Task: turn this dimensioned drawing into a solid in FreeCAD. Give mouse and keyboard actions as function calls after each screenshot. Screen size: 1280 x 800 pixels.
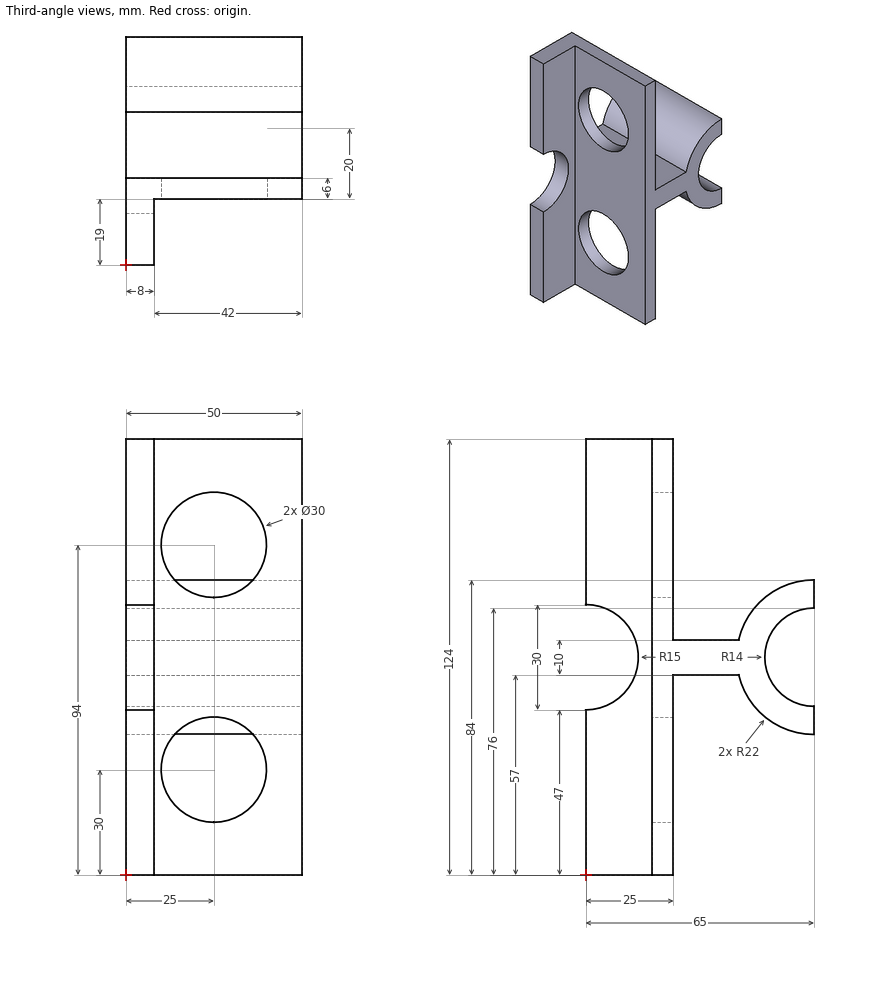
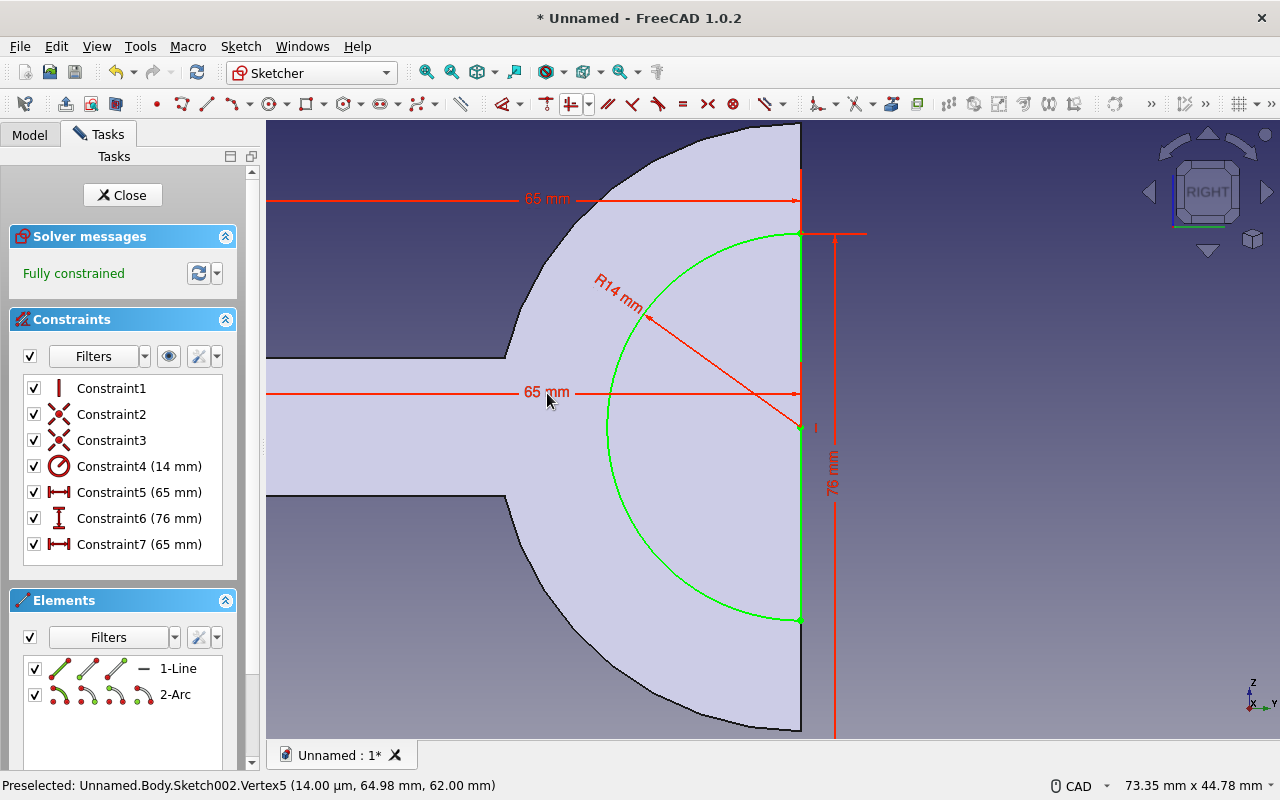
click(123, 195)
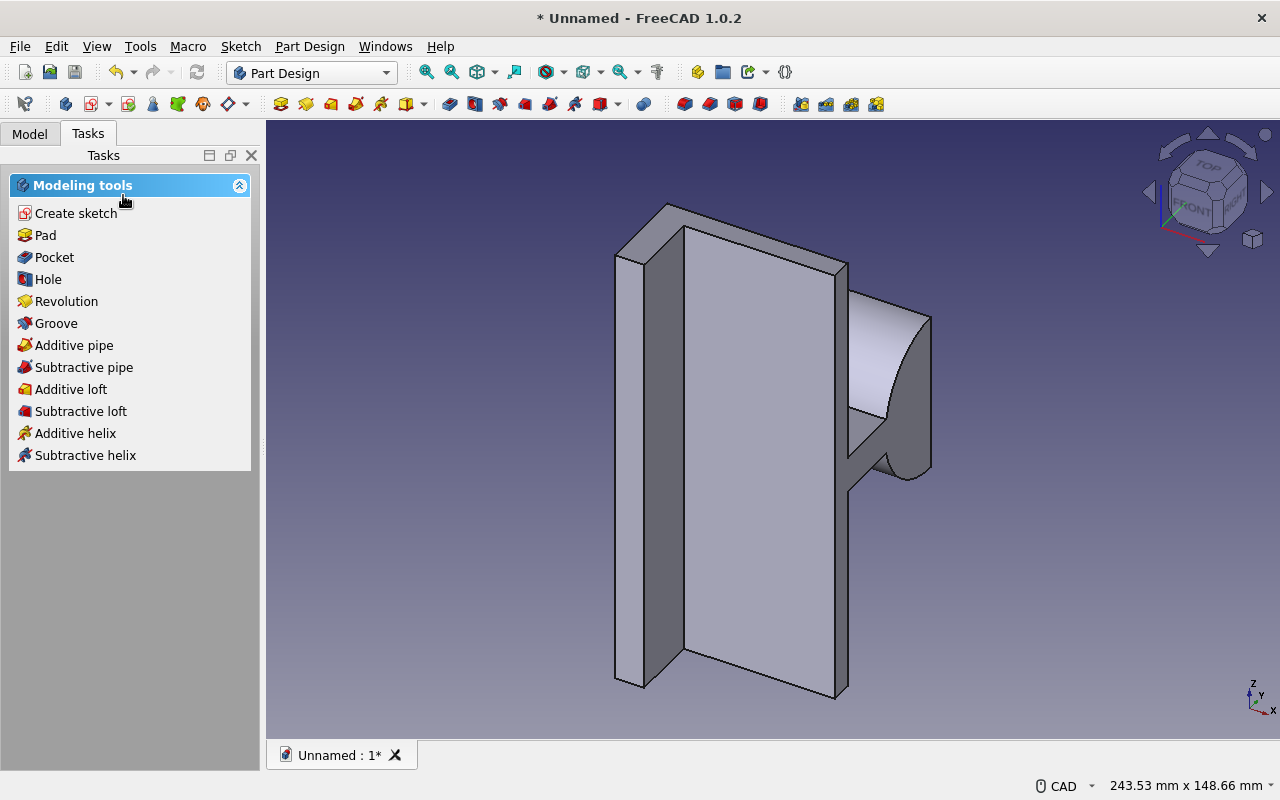
click(450, 104)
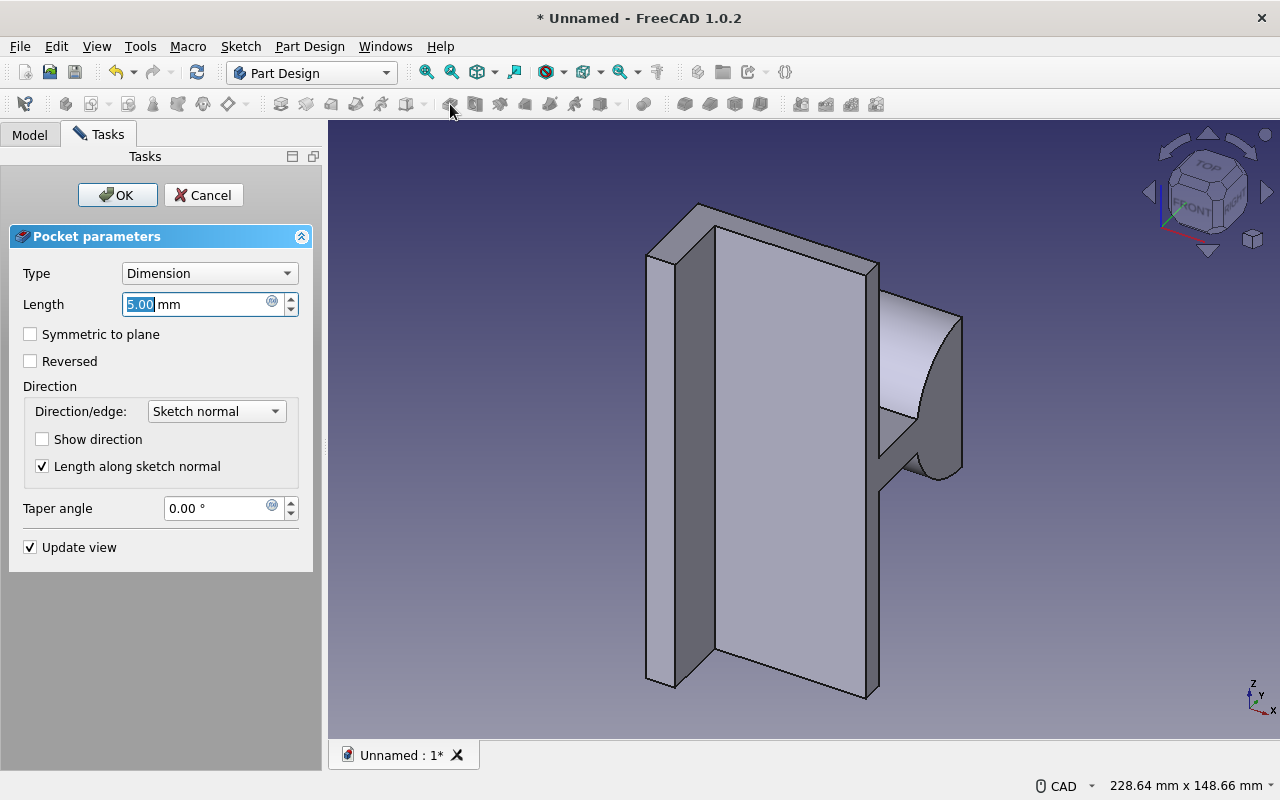
text(50)
key(Tab)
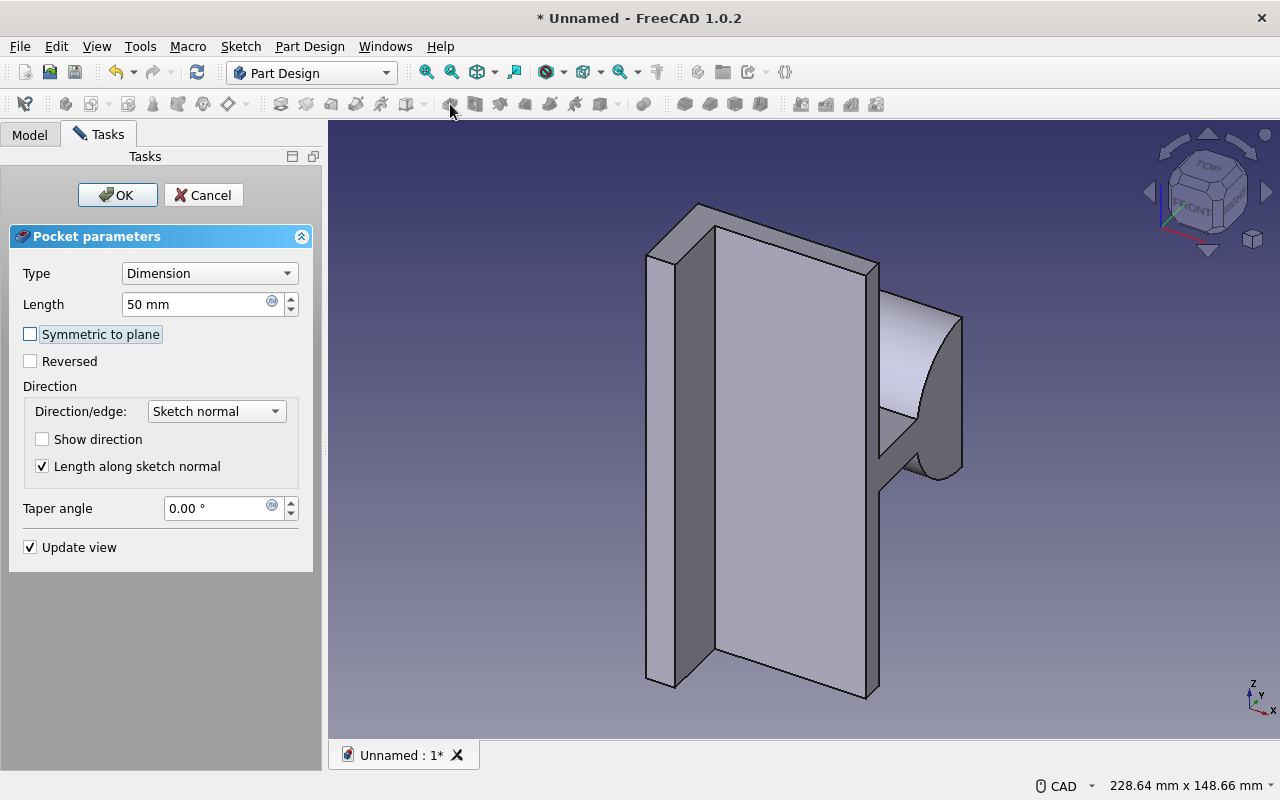
click(31, 361)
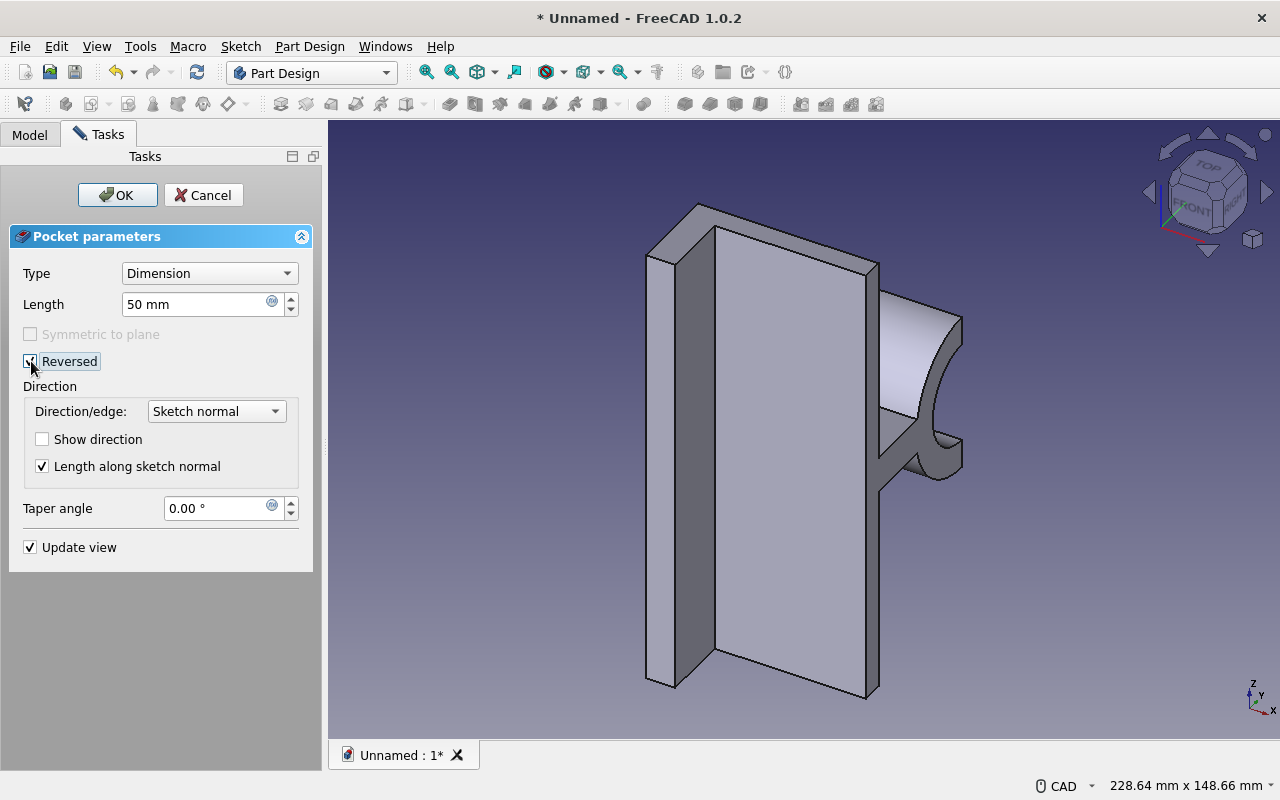
click(118, 195)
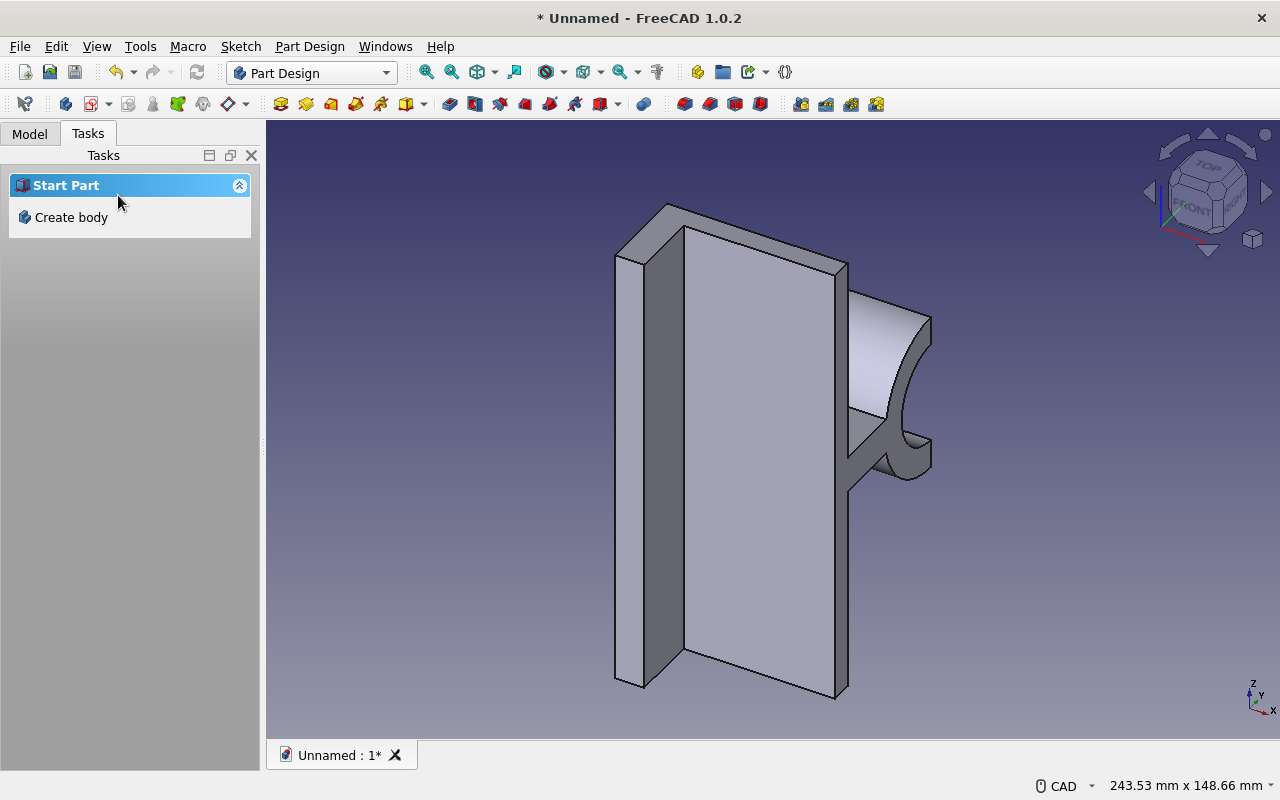
click(90, 104)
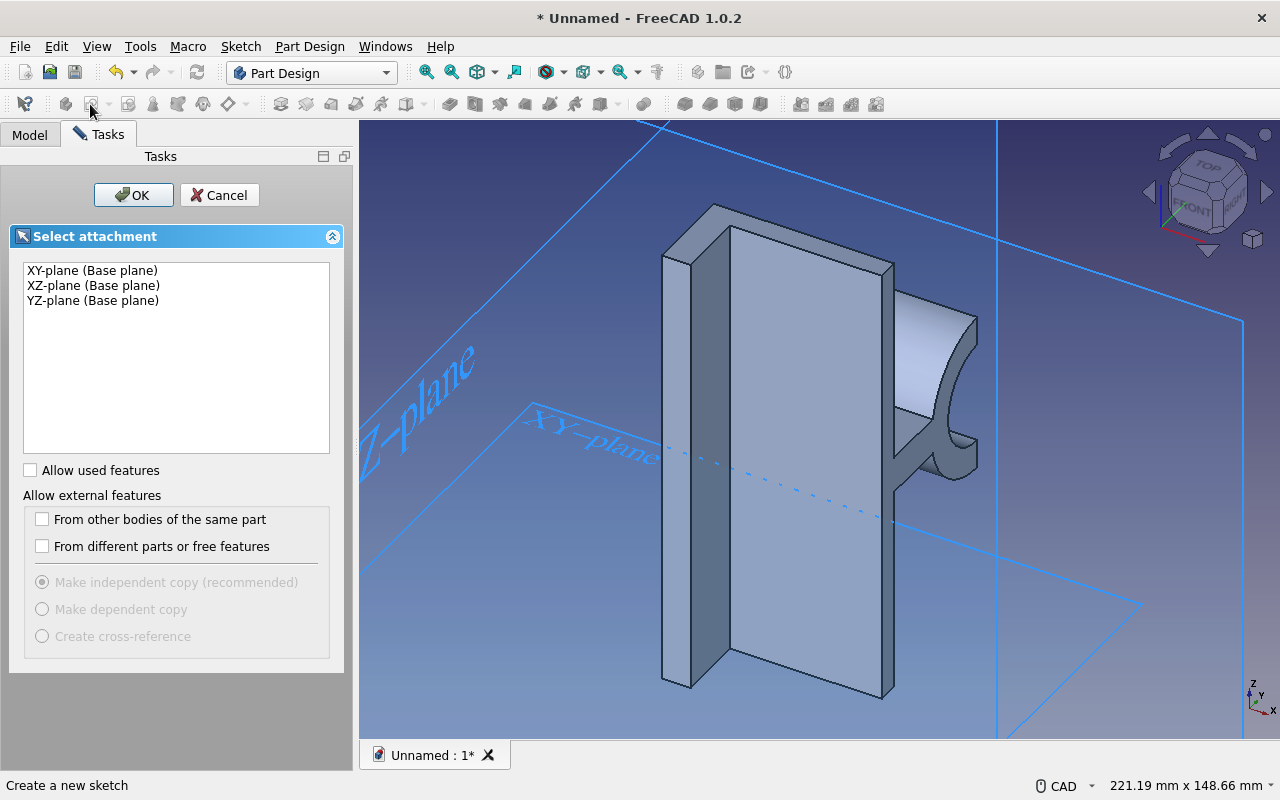
click(84, 300)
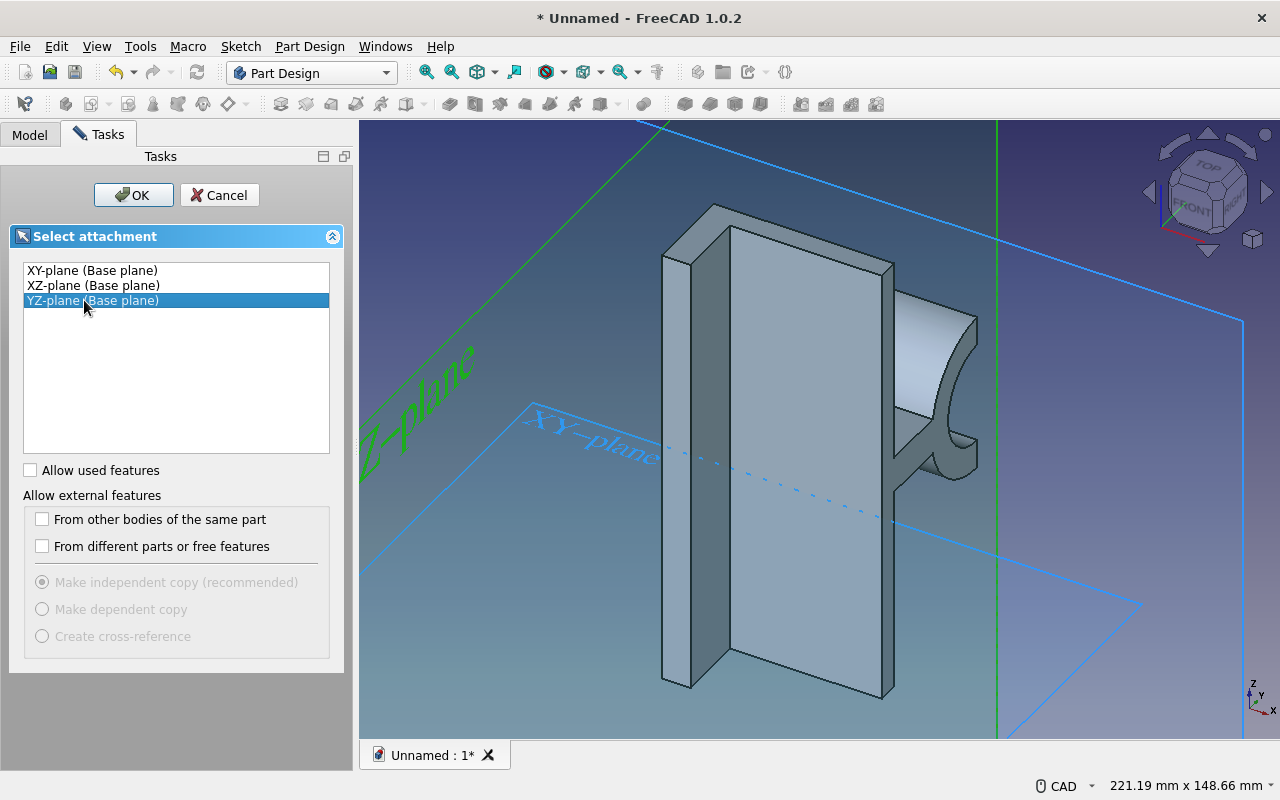
click(134, 195)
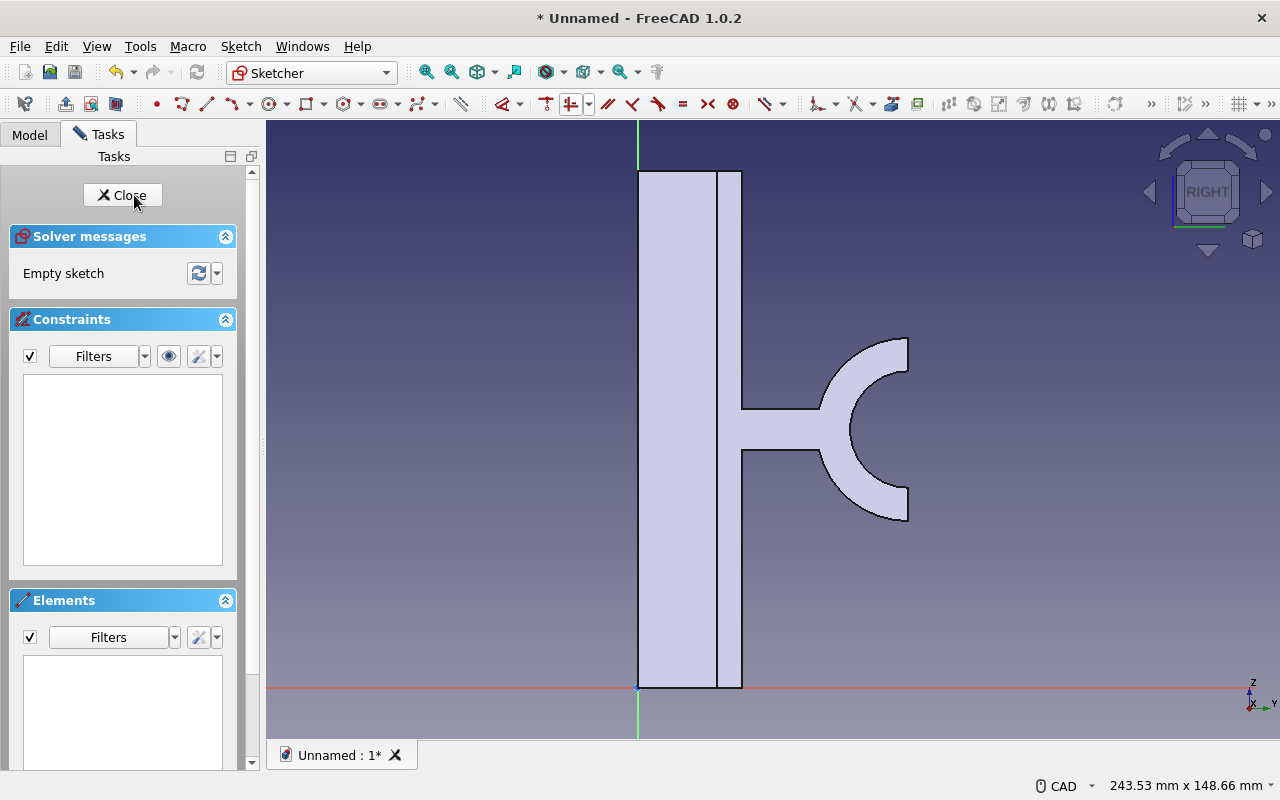
click(116, 104)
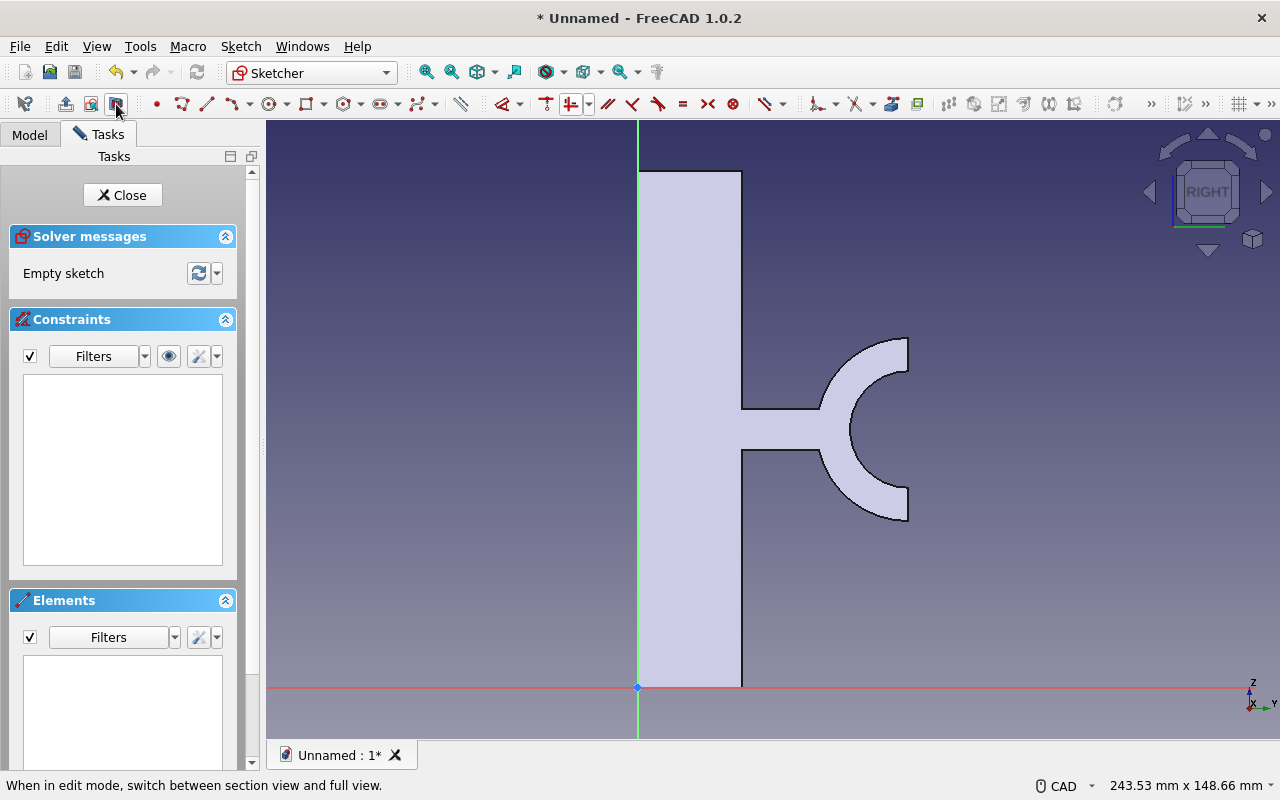
scroll(654, 430, up, 6)